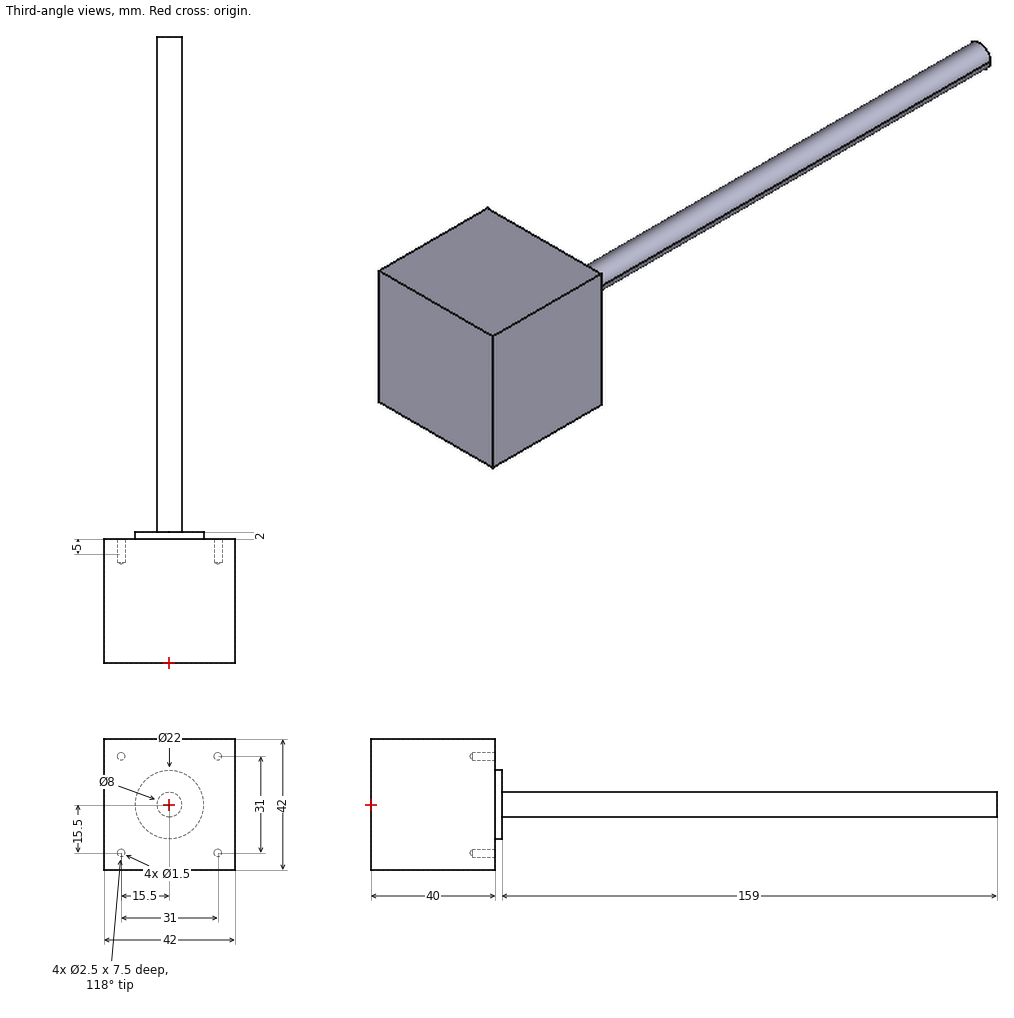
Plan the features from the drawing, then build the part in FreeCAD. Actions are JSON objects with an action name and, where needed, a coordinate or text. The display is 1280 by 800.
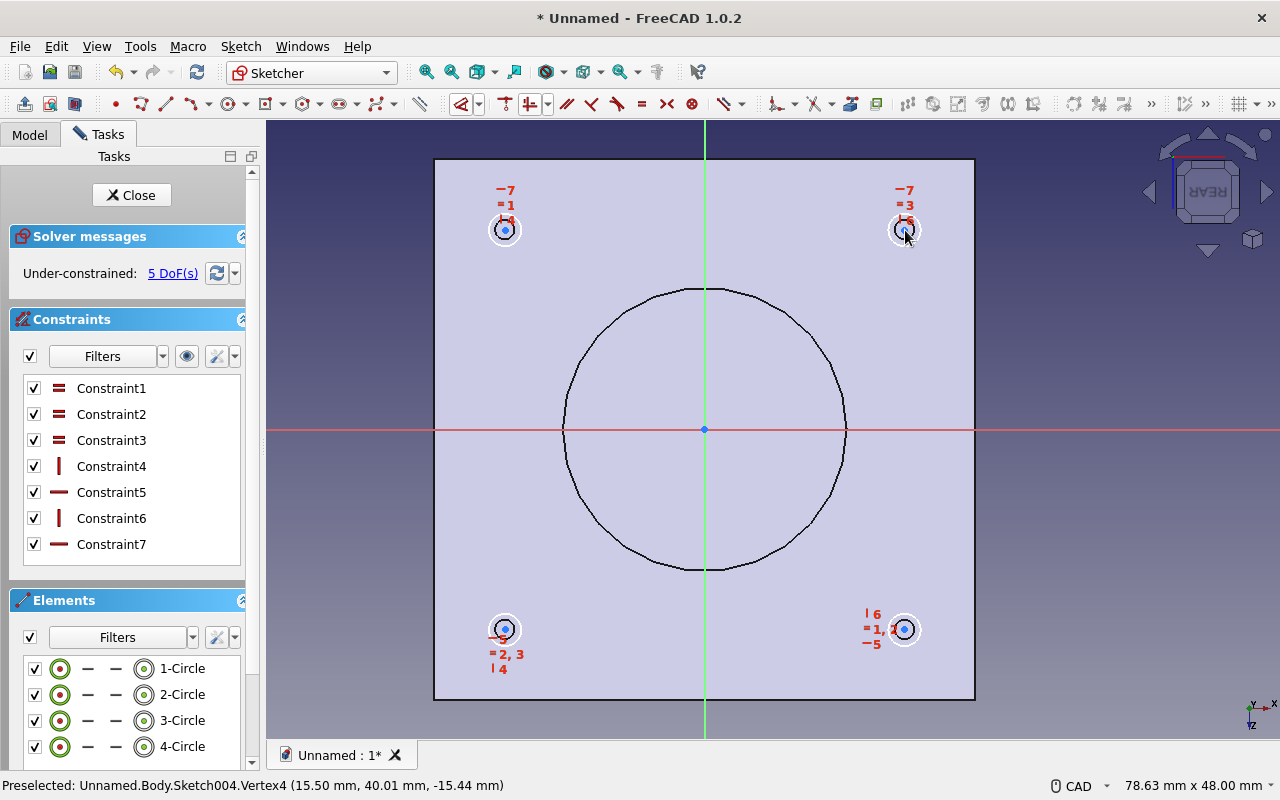
{"action": "scroll", "coordinate": [516, 219], "scroll_direction": "up", "scroll_amount": 2}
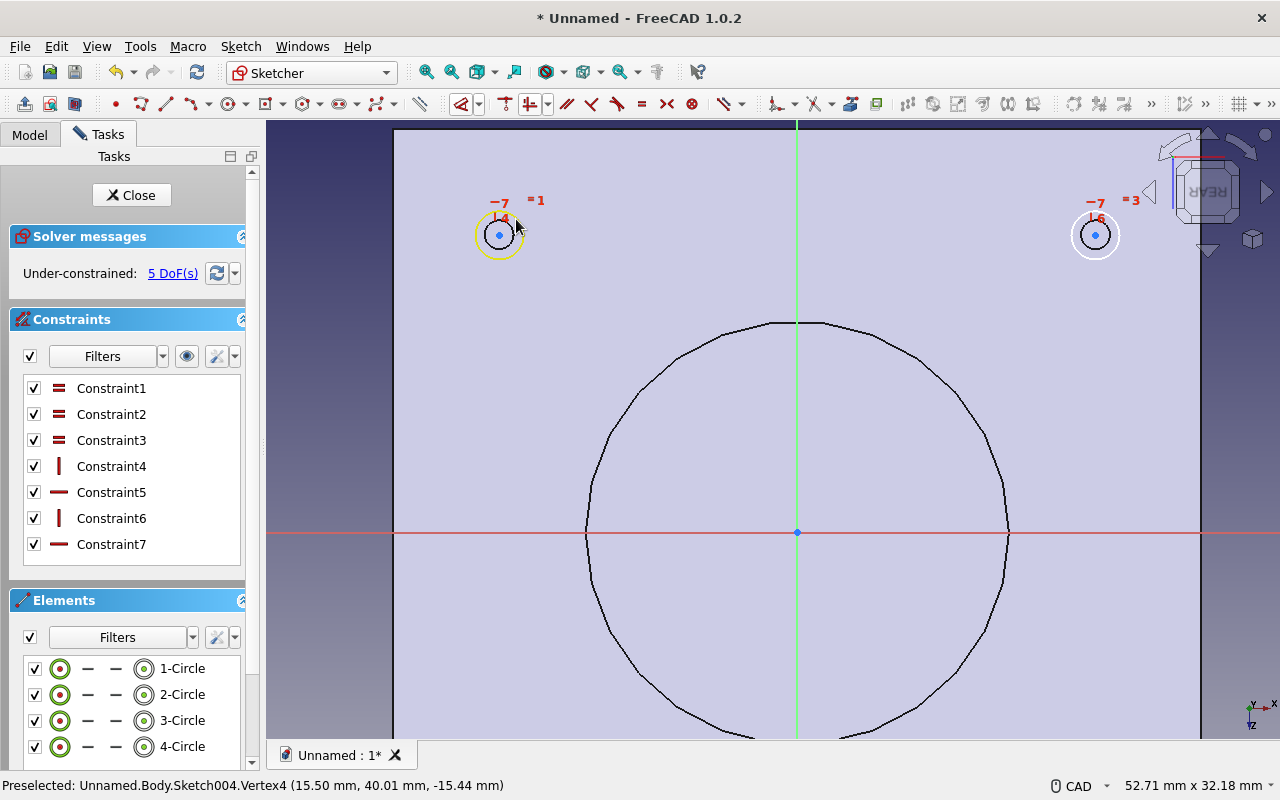
{"action": "left_click", "coordinate": [517, 218]}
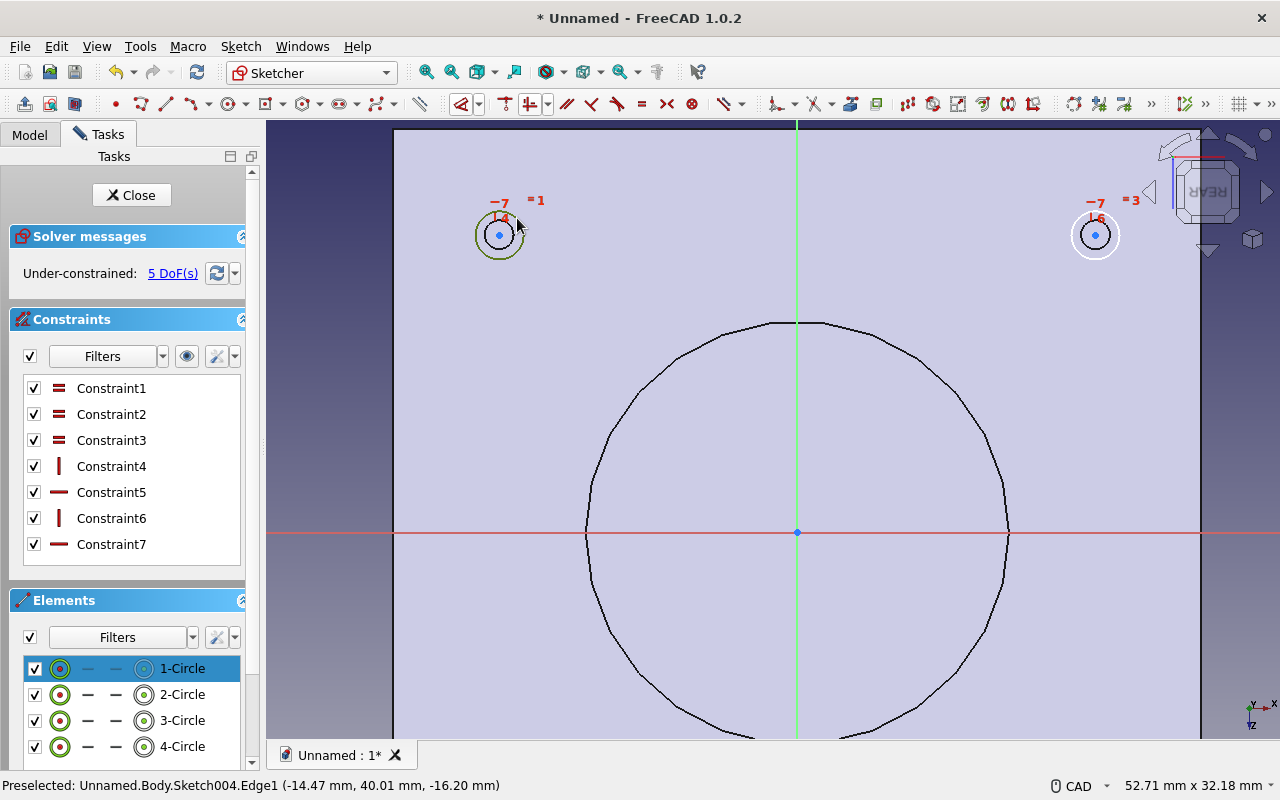
{"action": "key", "text": "k o"}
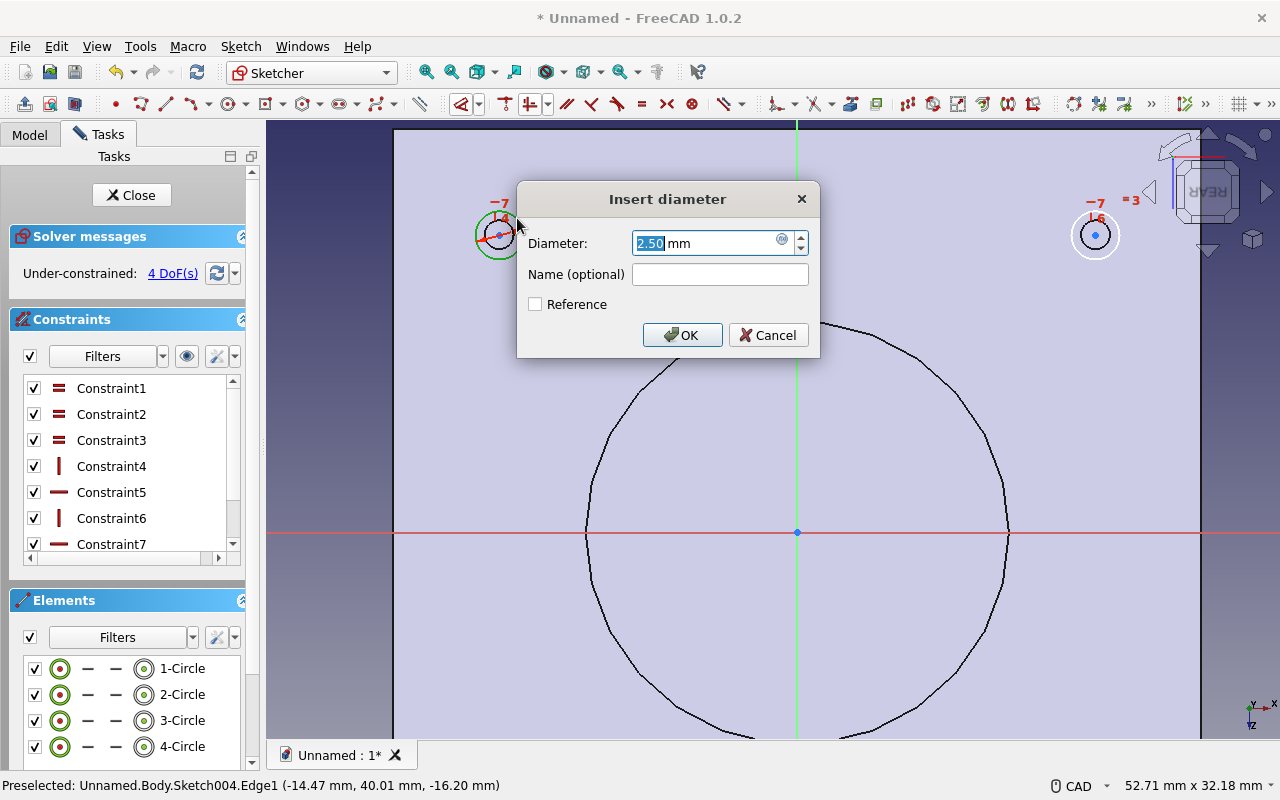
{"action": "type", "text": "2.5"}
{"action": "key", "text": "Return"}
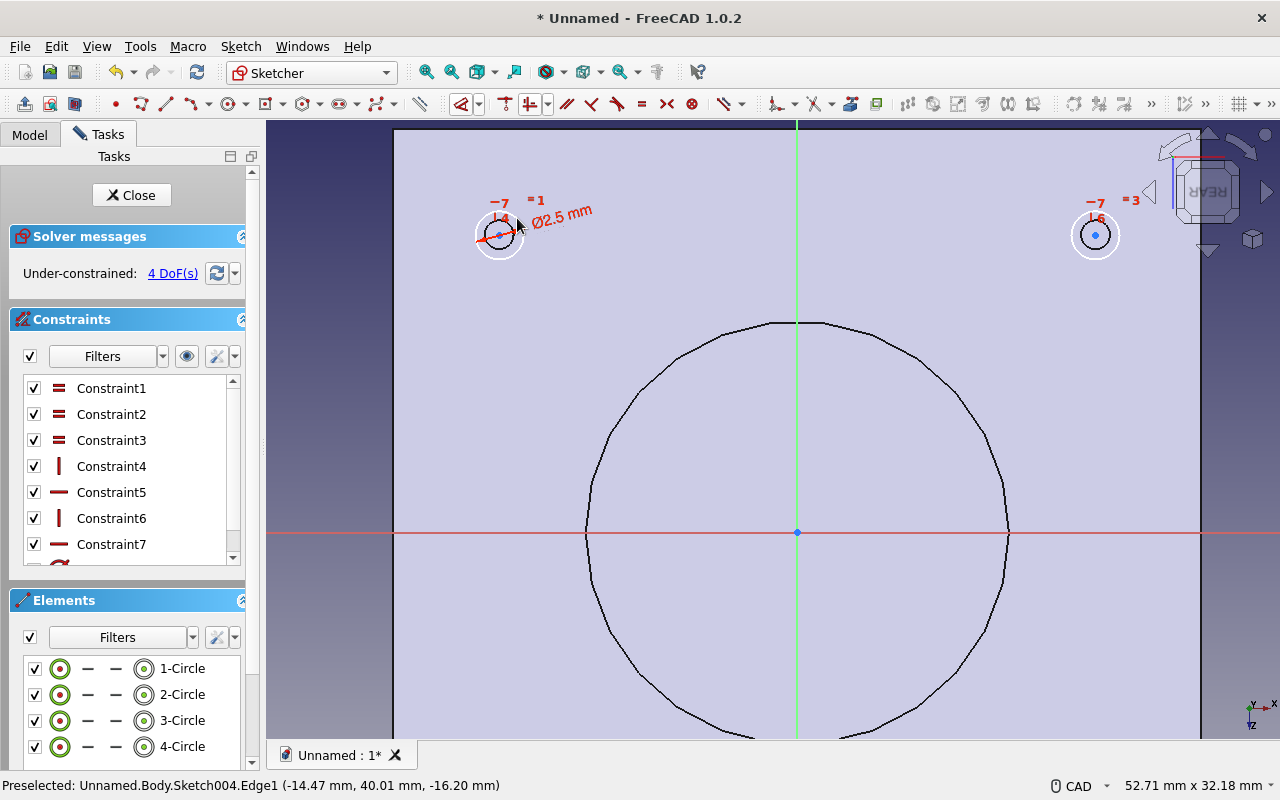
{"action": "left_click", "coordinate": [500, 235]}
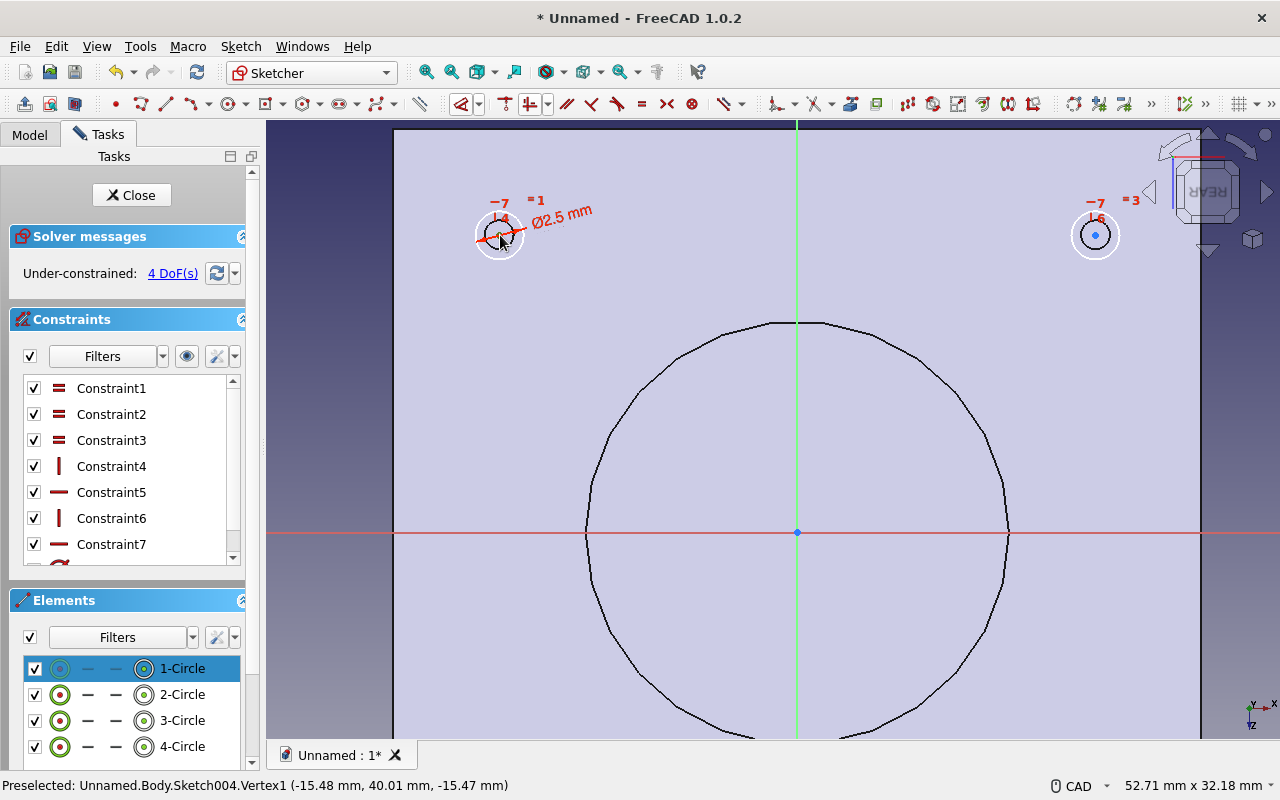
{"action": "scroll", "coordinate": [516, 219], "scroll_direction": "down", "scroll_amount": 2}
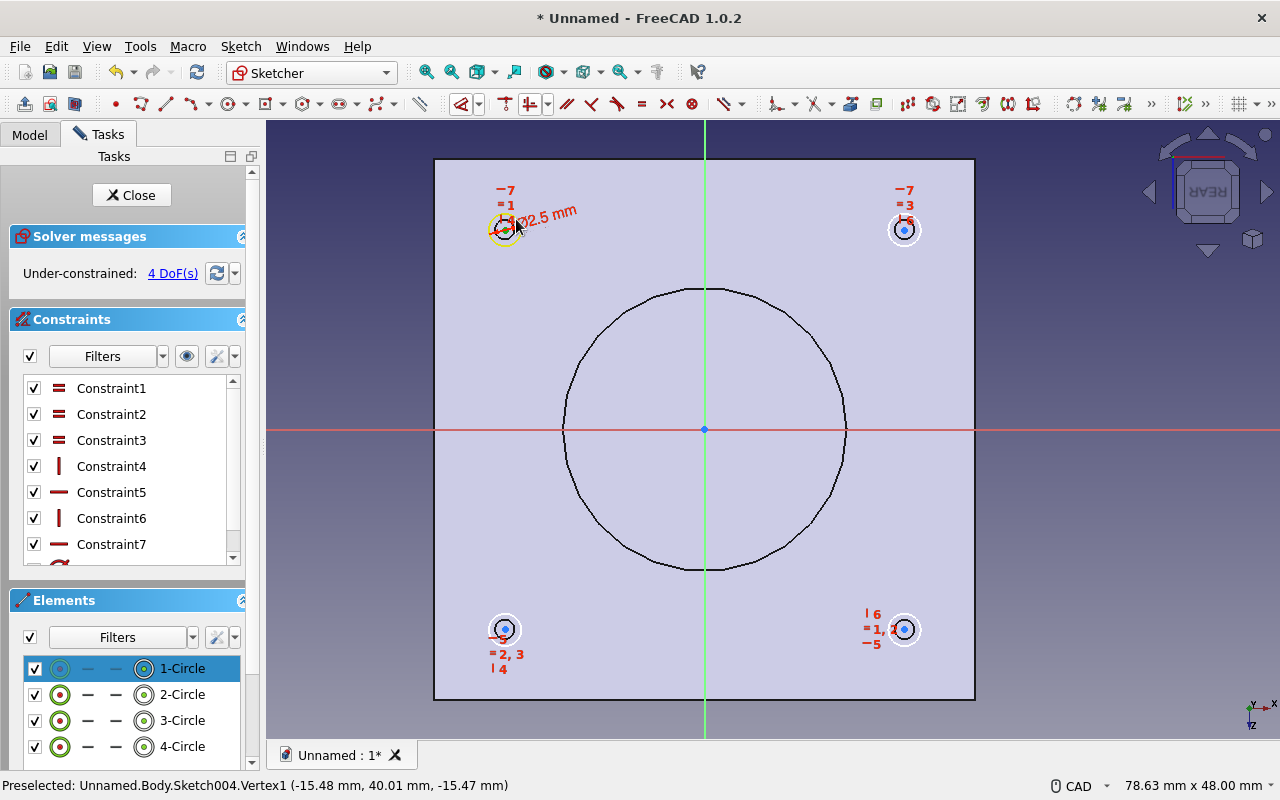
{"action": "left_click", "coordinate": [905, 630]}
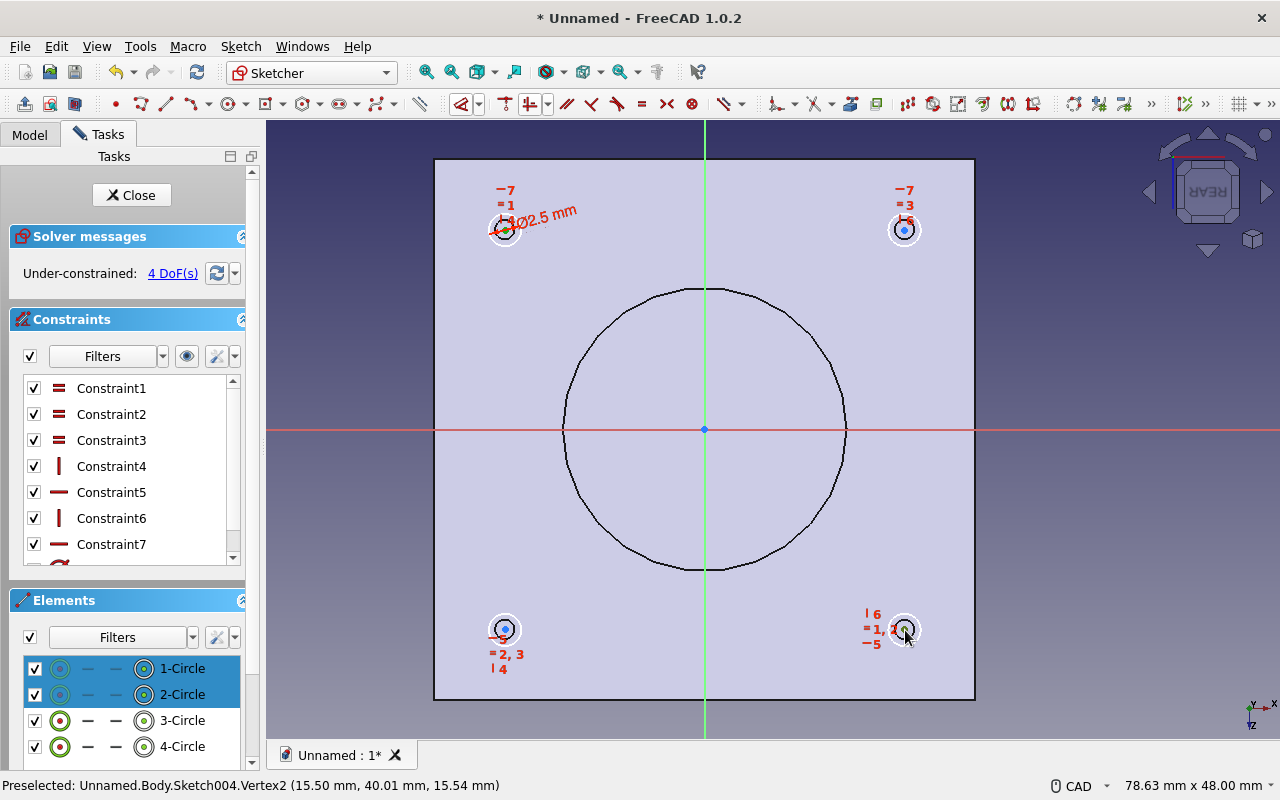
{"action": "key", "text": "l"}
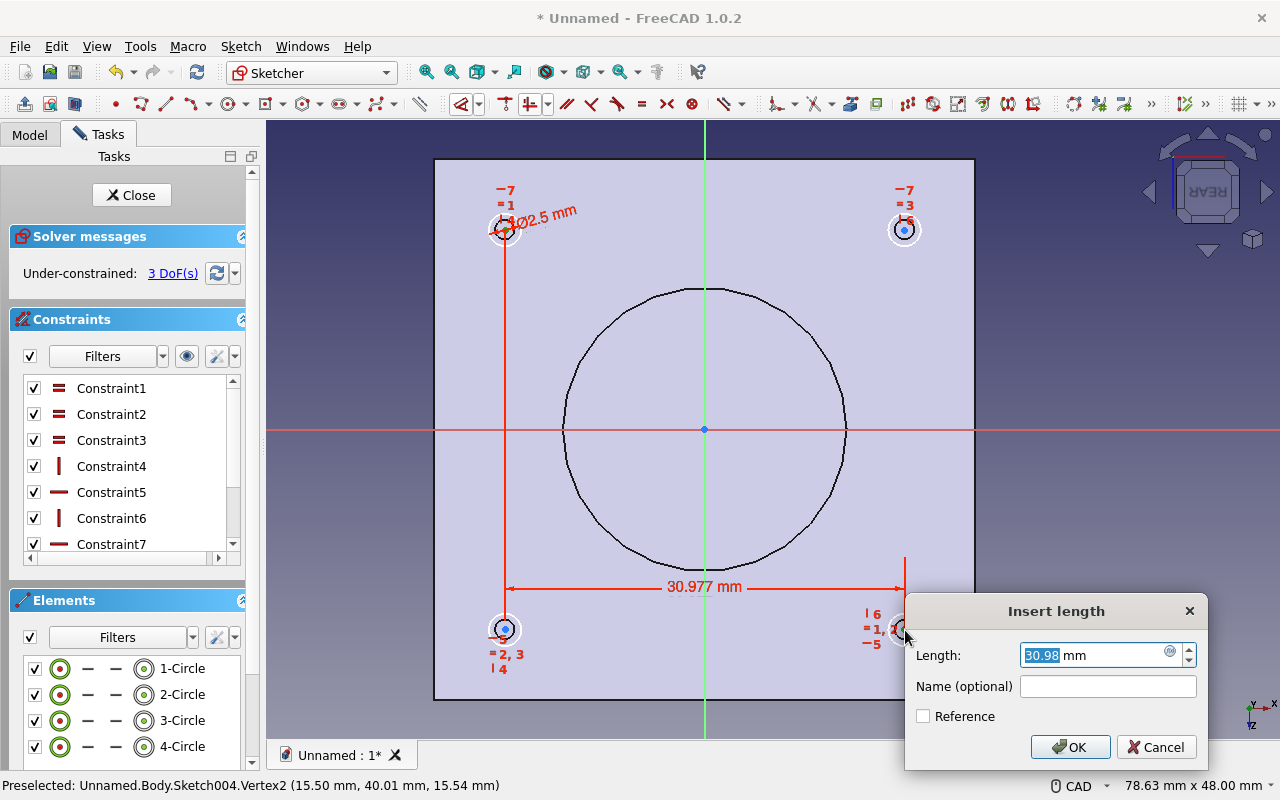
{"action": "type", "text": "31"}
{"action": "key", "text": "Return"}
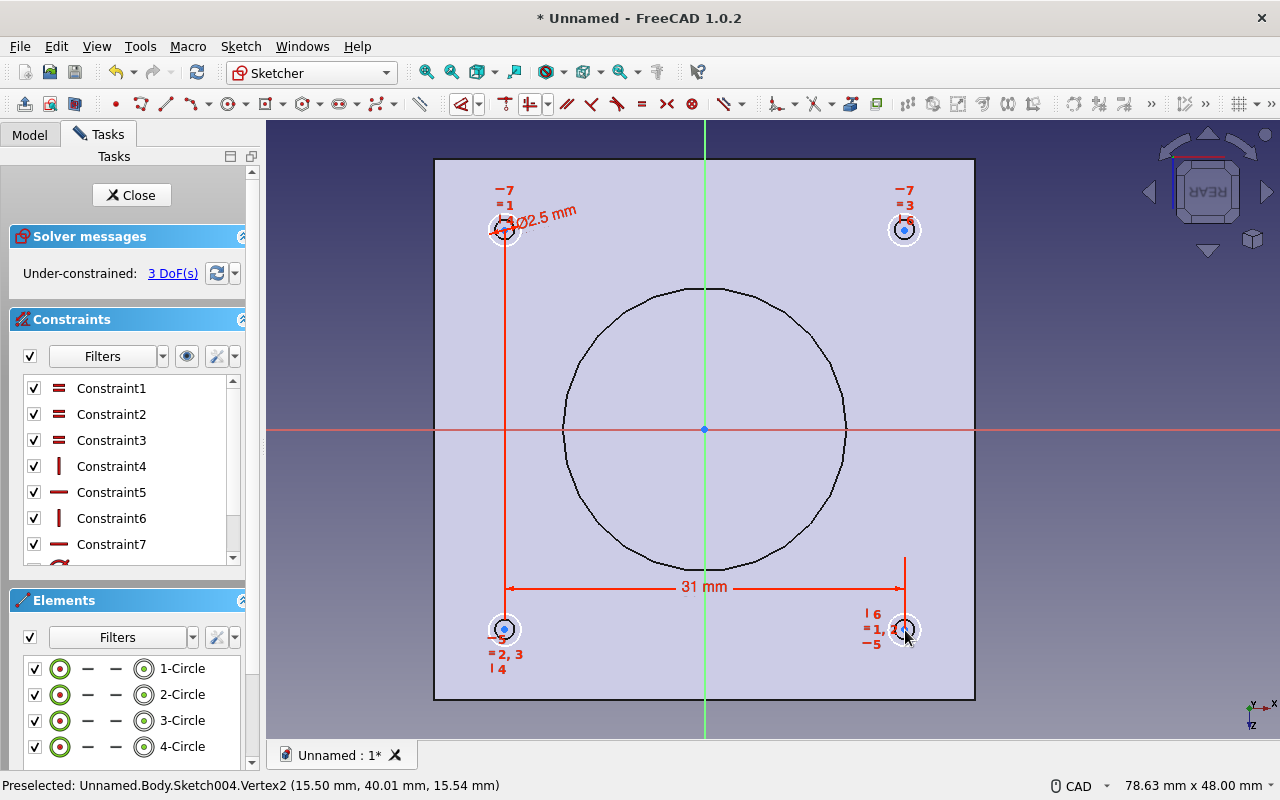
{"action": "left_click", "coordinate": [505, 230]}